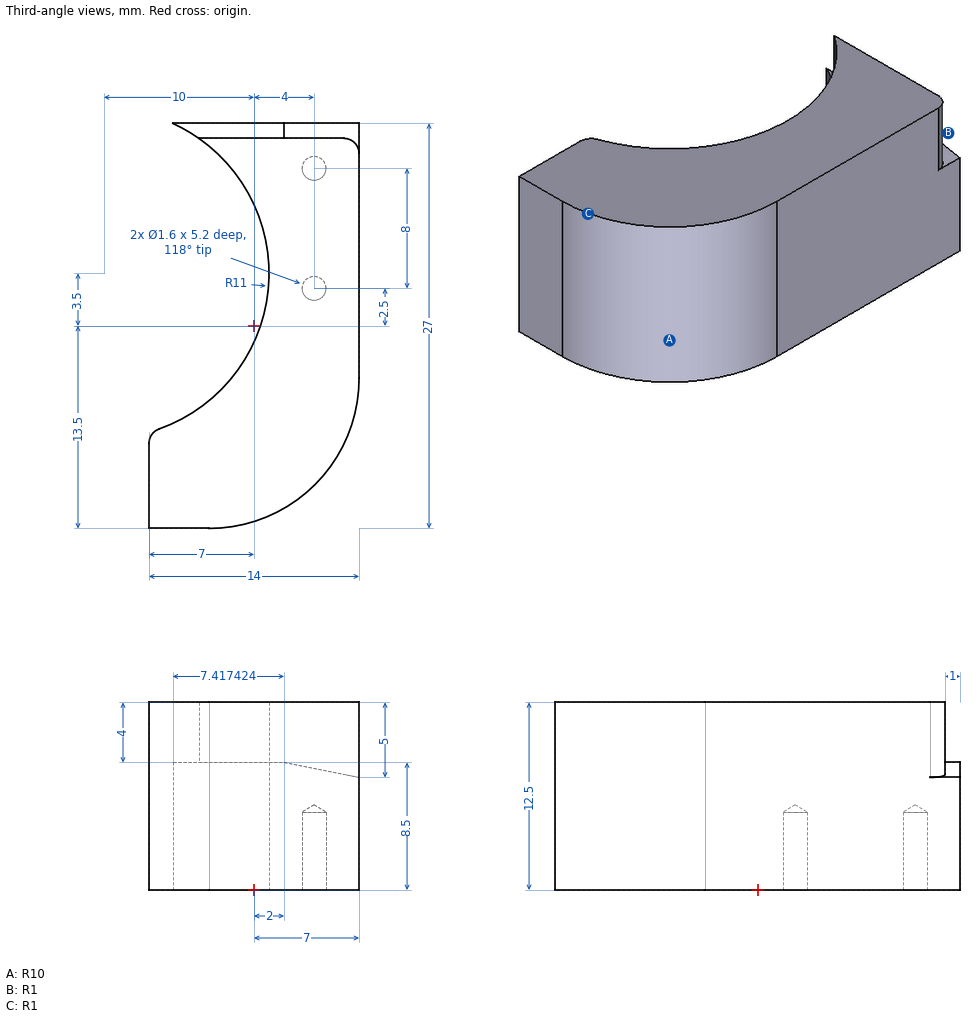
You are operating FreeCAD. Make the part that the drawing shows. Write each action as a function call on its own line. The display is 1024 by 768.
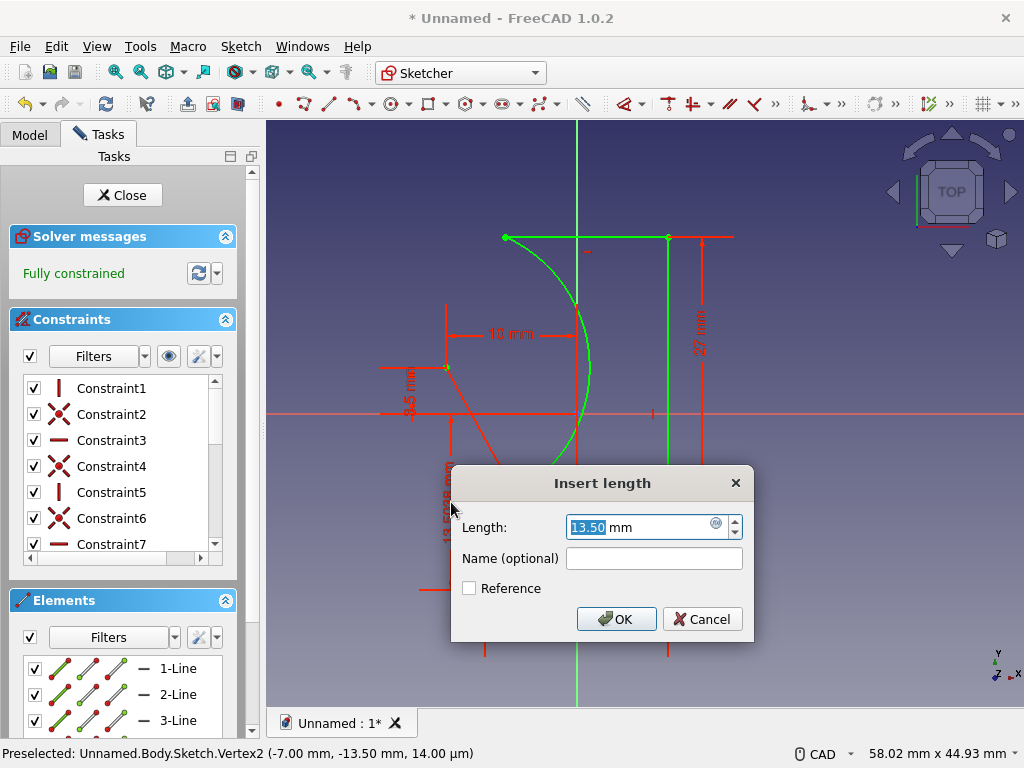
text(13.5)
key(Return)
key(Escape)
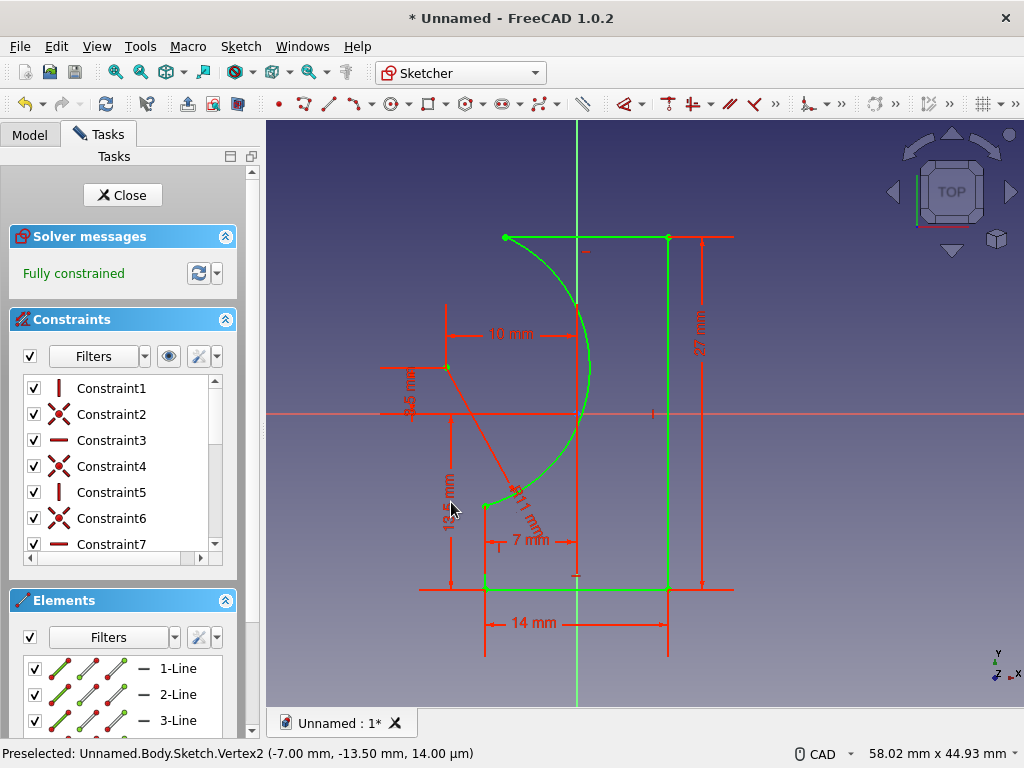
click(123, 195)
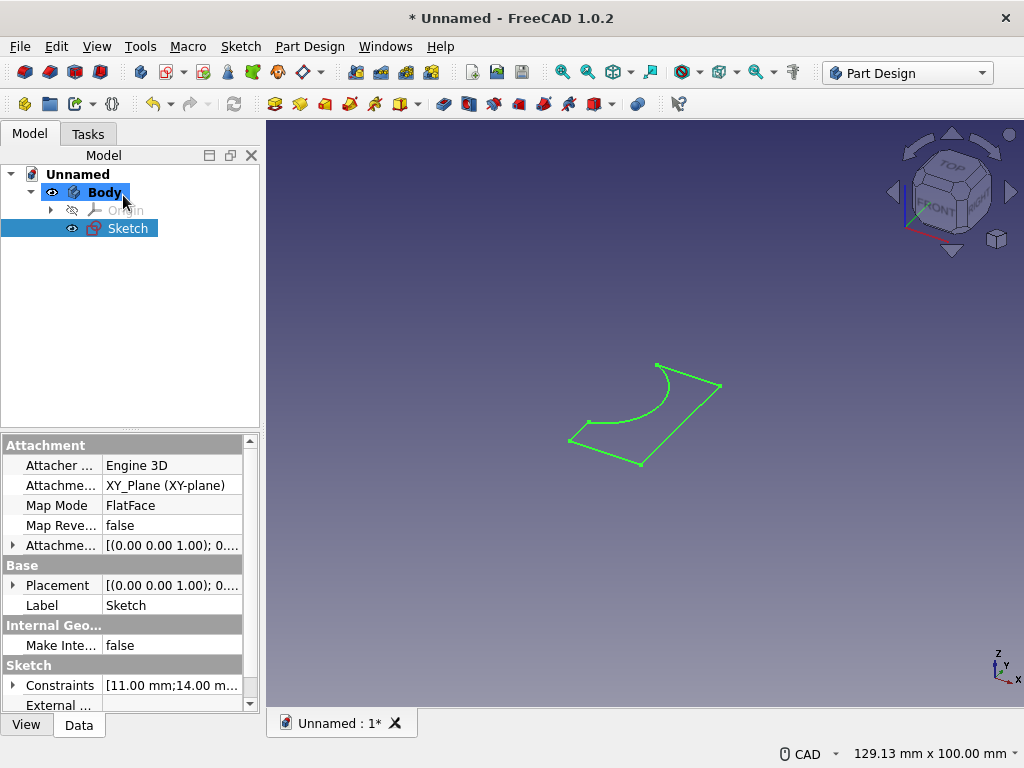
click(275, 104)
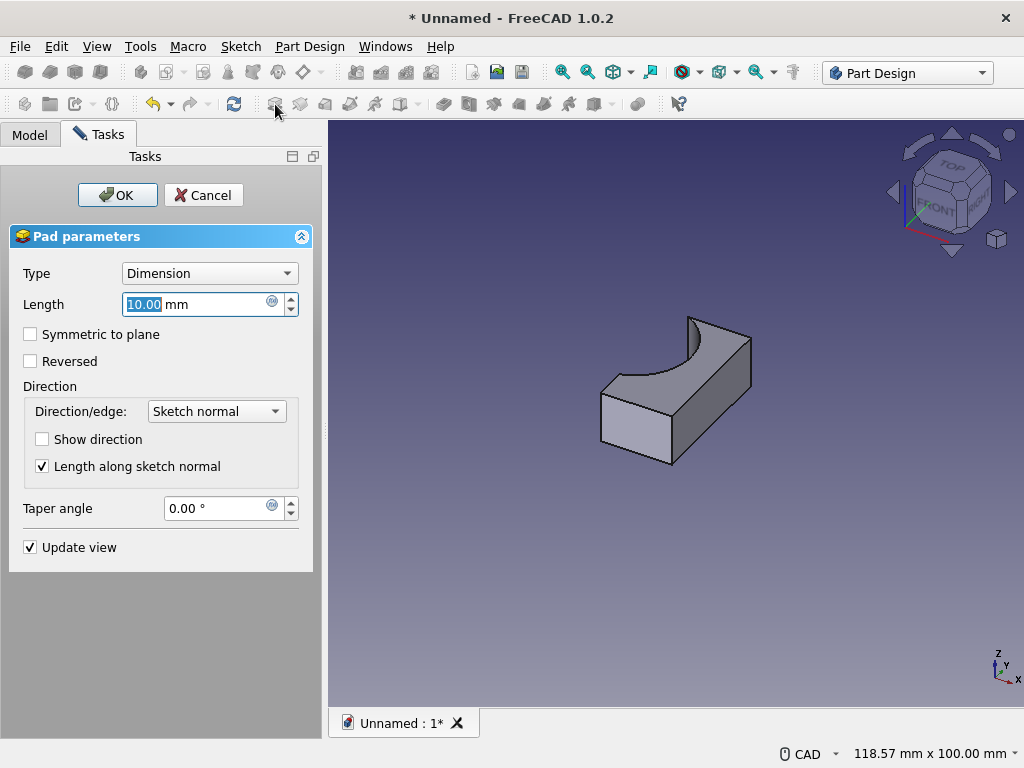
text(12.5)
key(Tab)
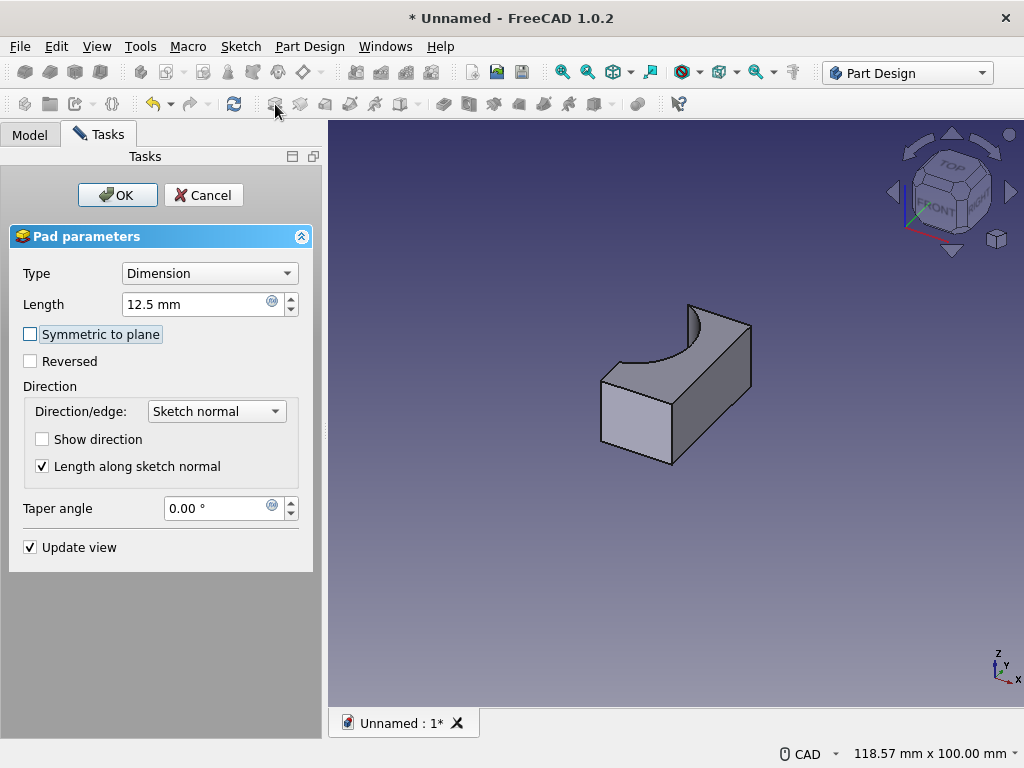
click(118, 195)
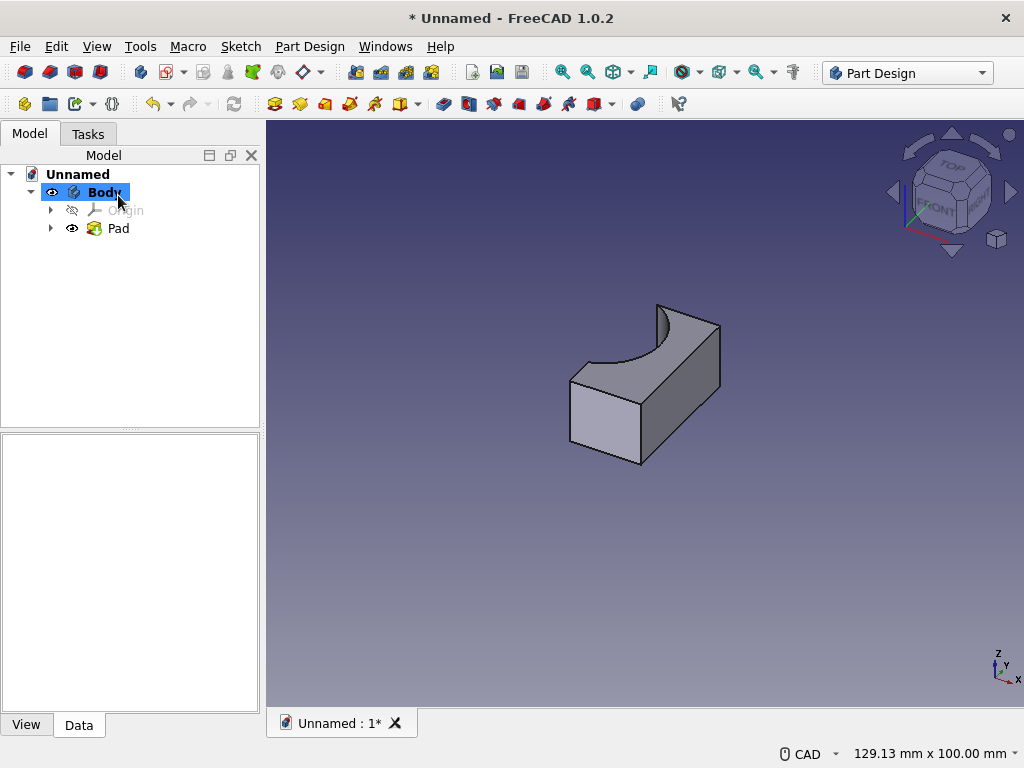
click(563, 72)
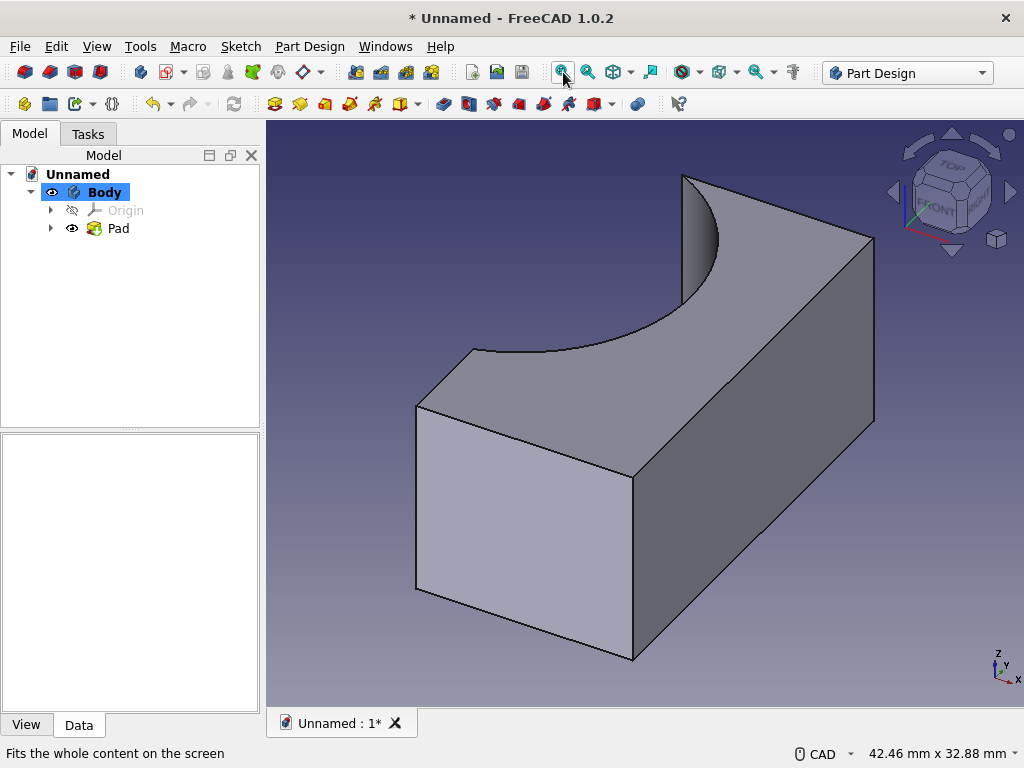
key(4)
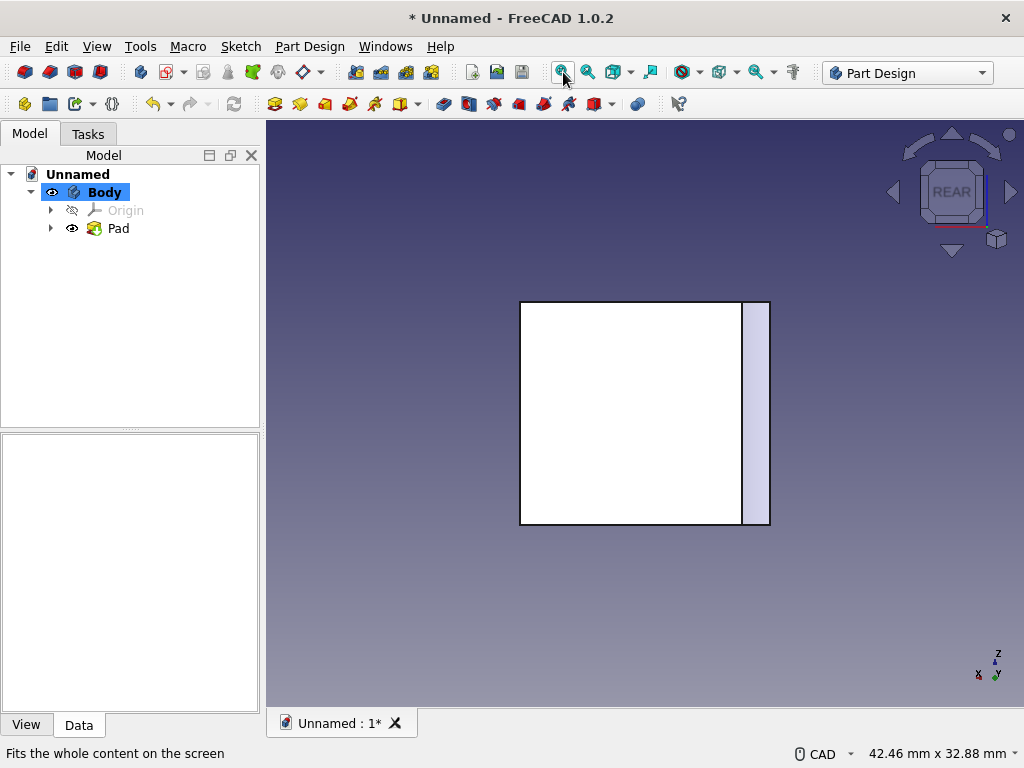
click(563, 72)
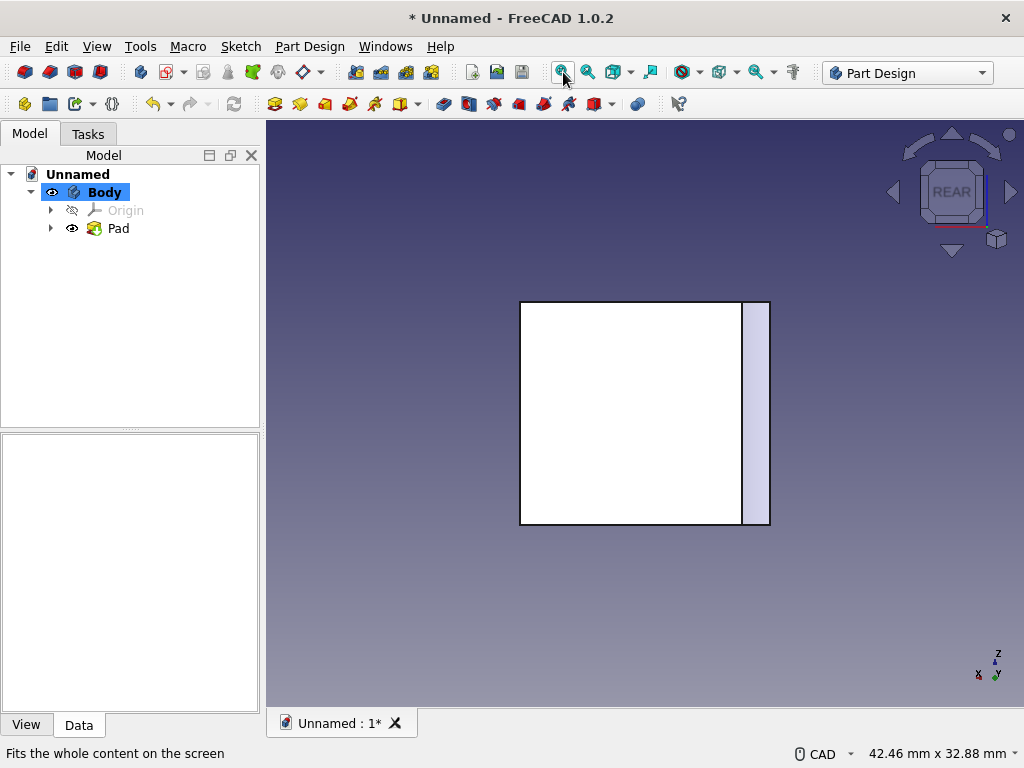
click(631, 413)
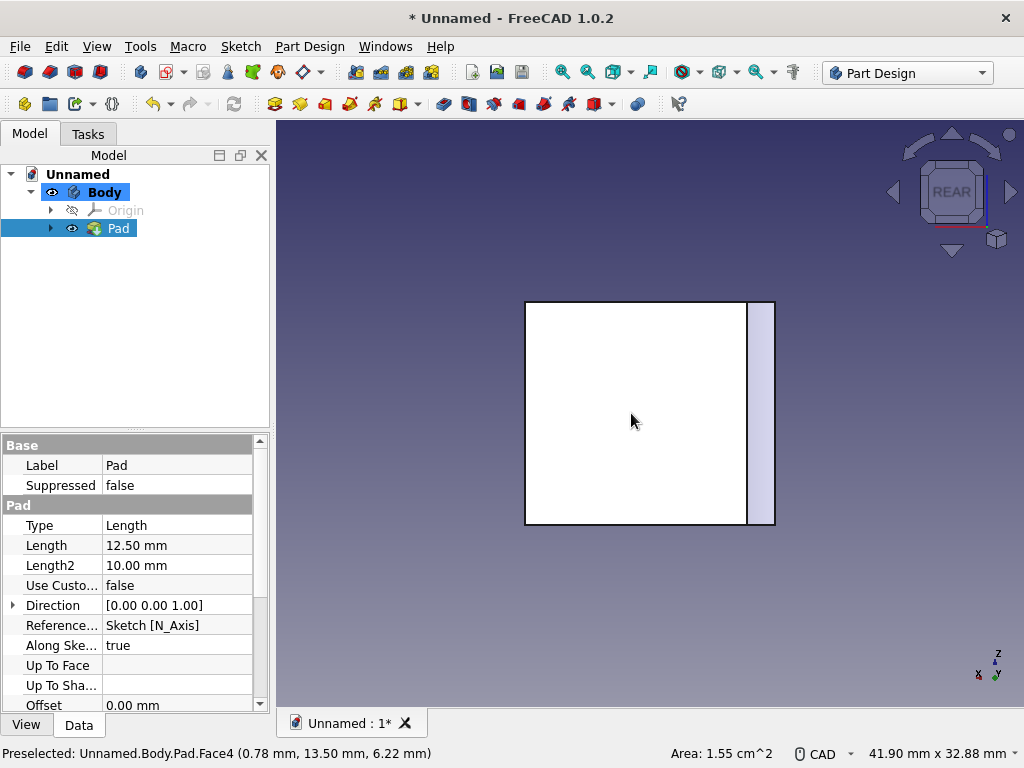
click(166, 72)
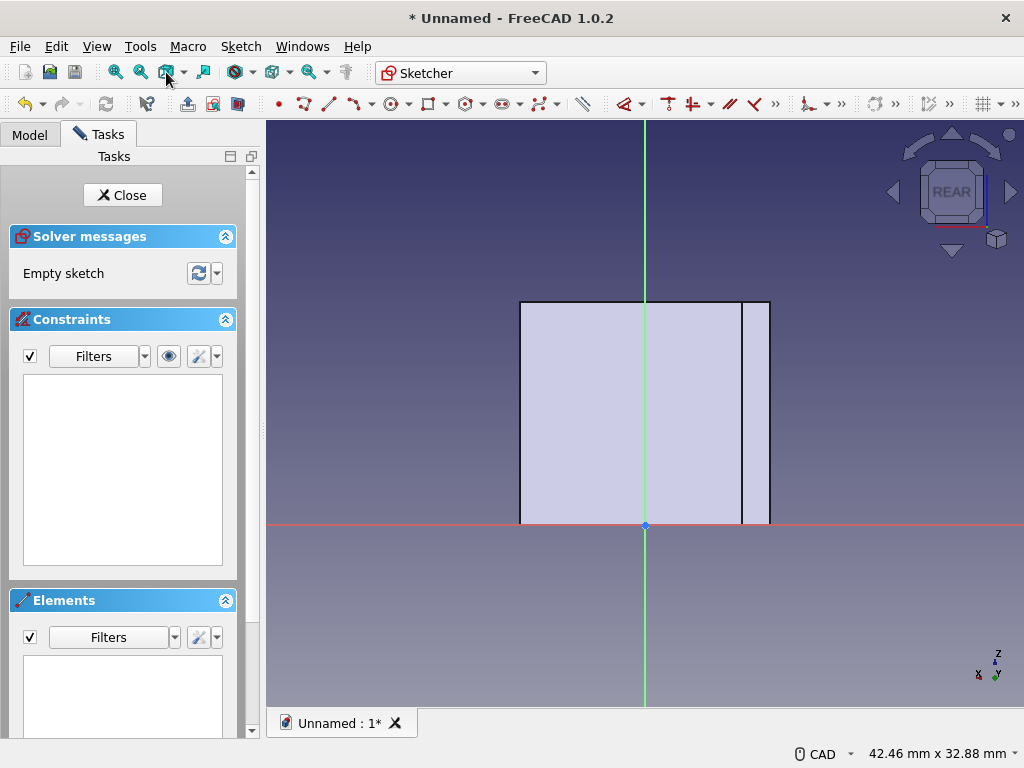
scroll(697, 414, up, 3)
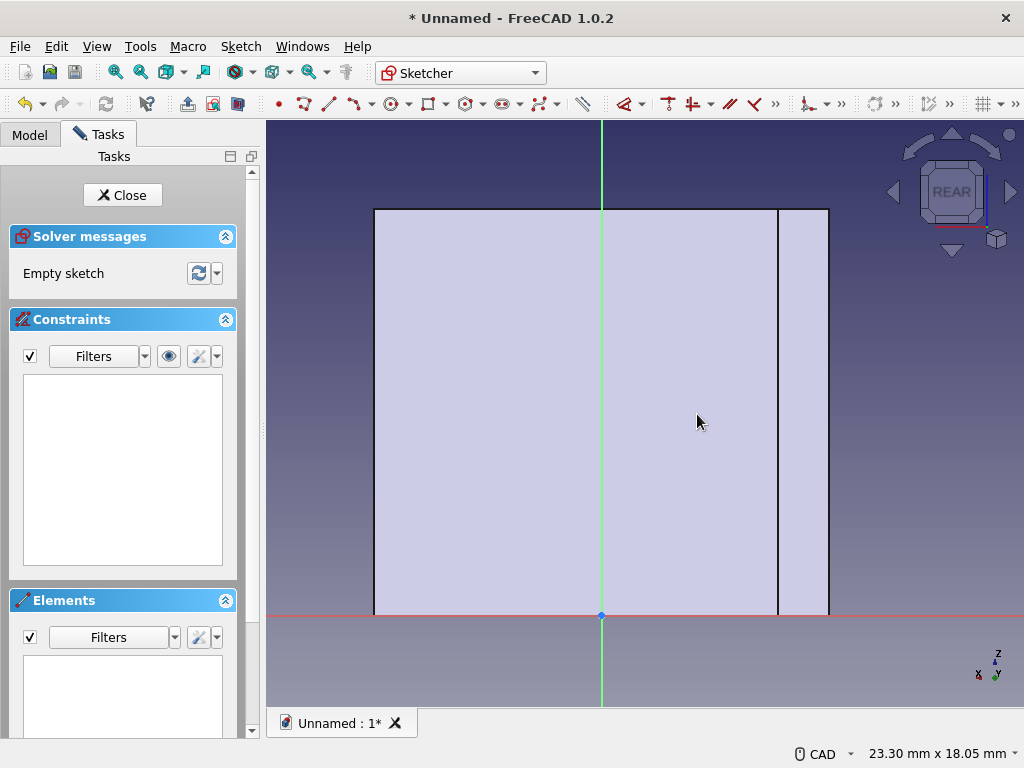
click(304, 104)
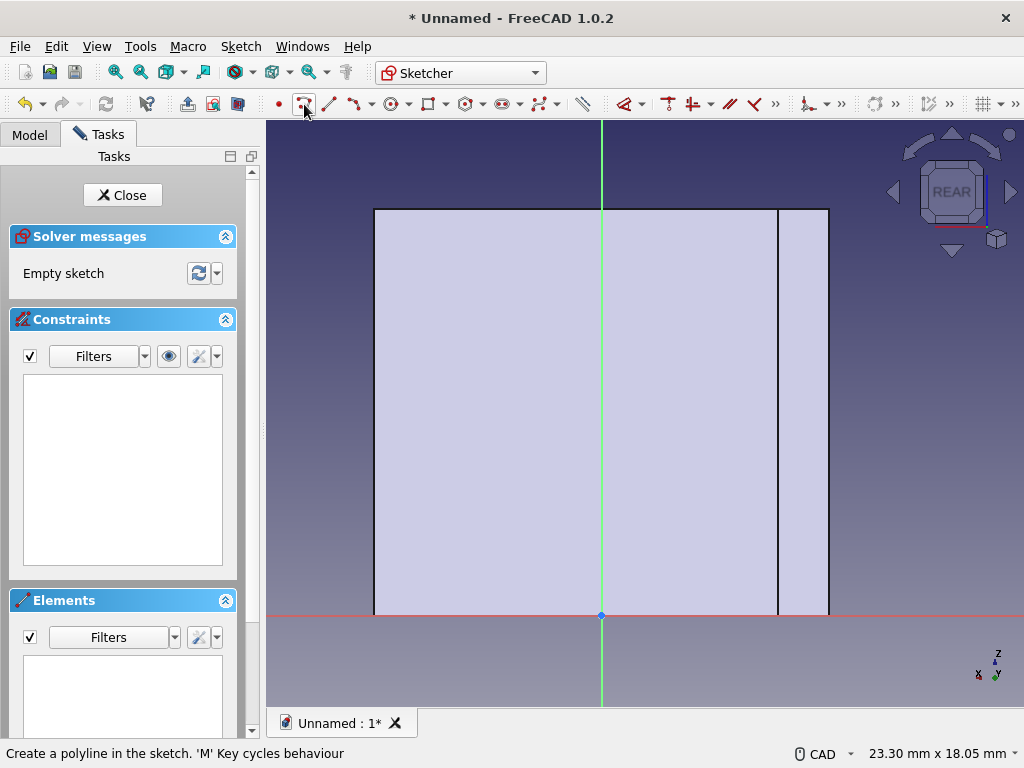
click(537, 339)
click(778, 339)
click(778, 209)
click(374, 209)
click(374, 372)
click(537, 340)
key(Escape)
key(Escape)